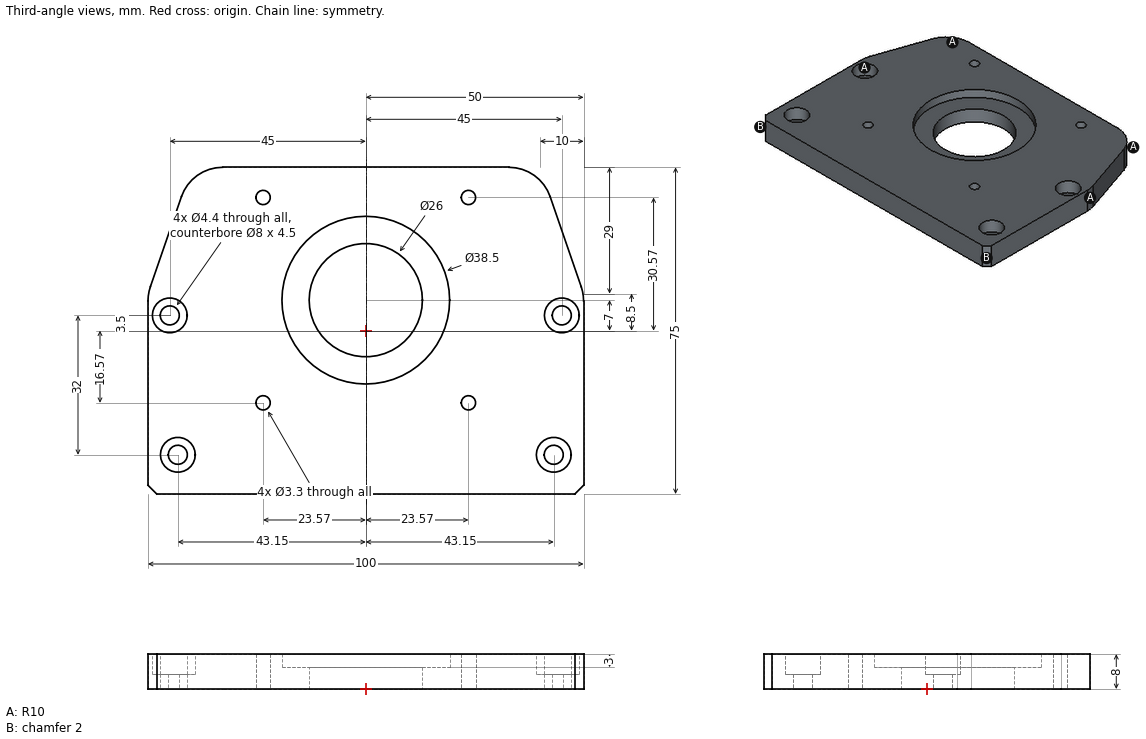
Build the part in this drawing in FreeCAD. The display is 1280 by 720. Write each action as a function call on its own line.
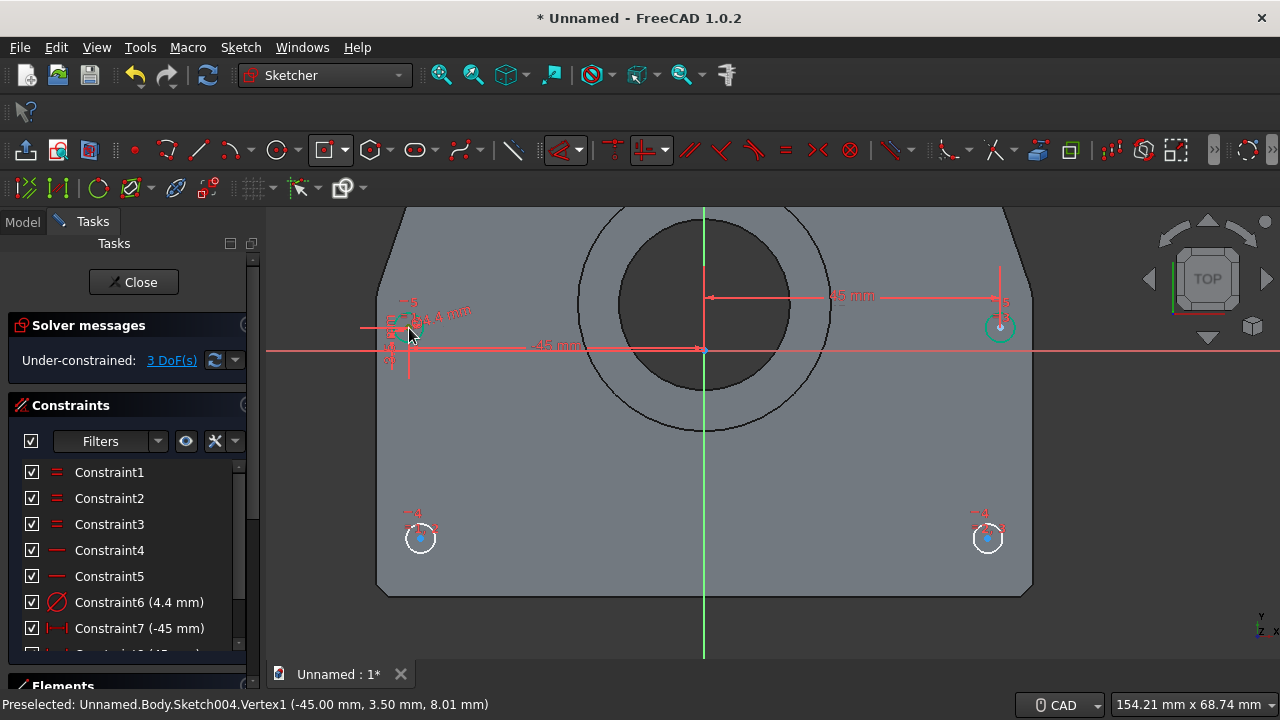
click(421, 539)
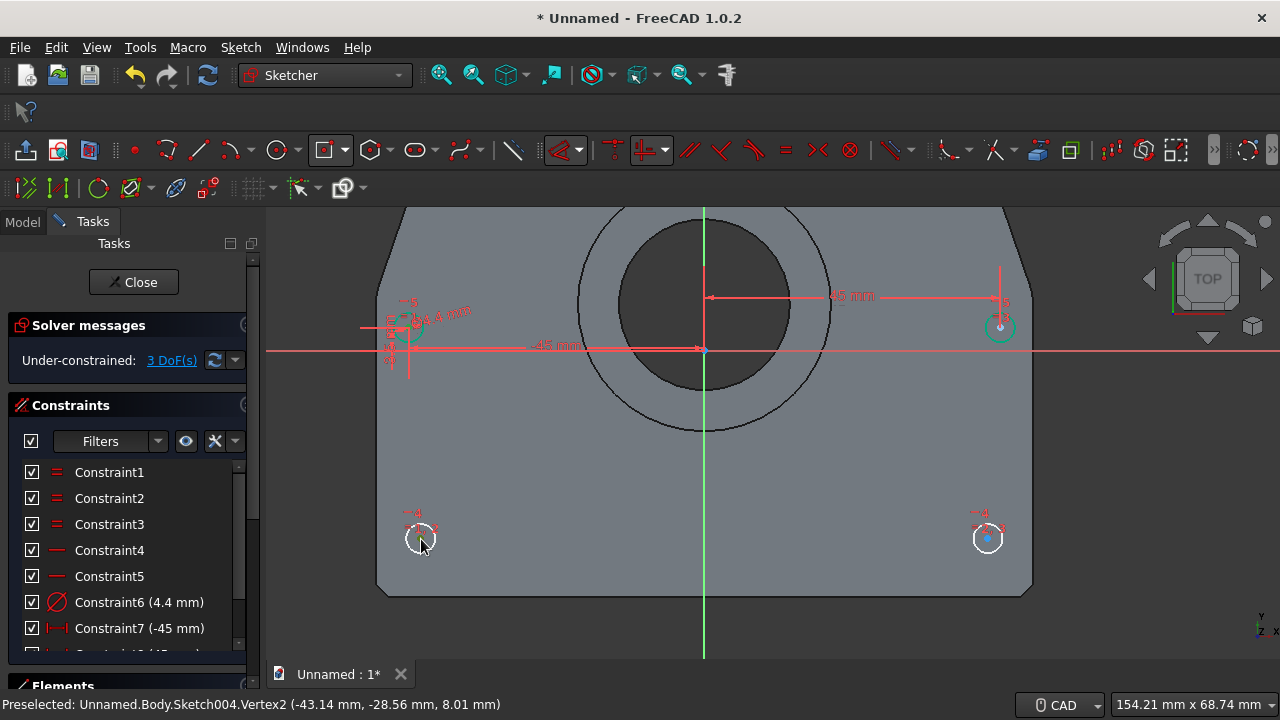
key(i)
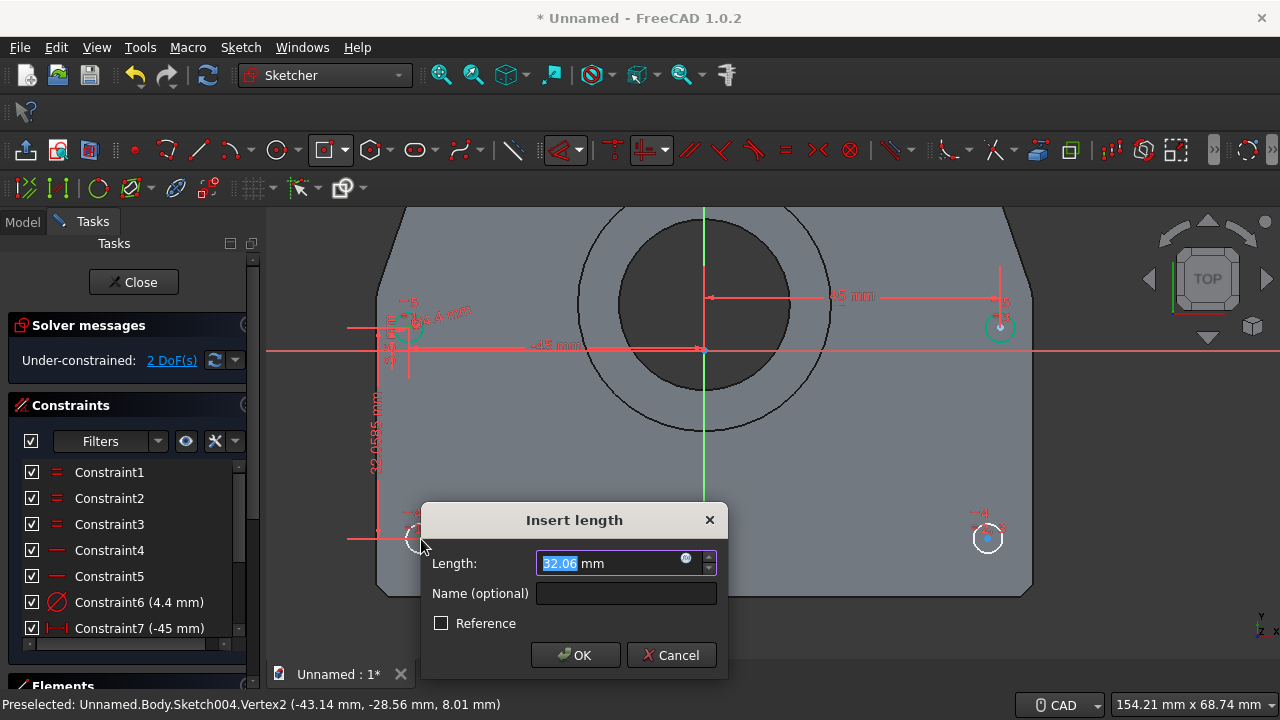
text(32)
key(Return)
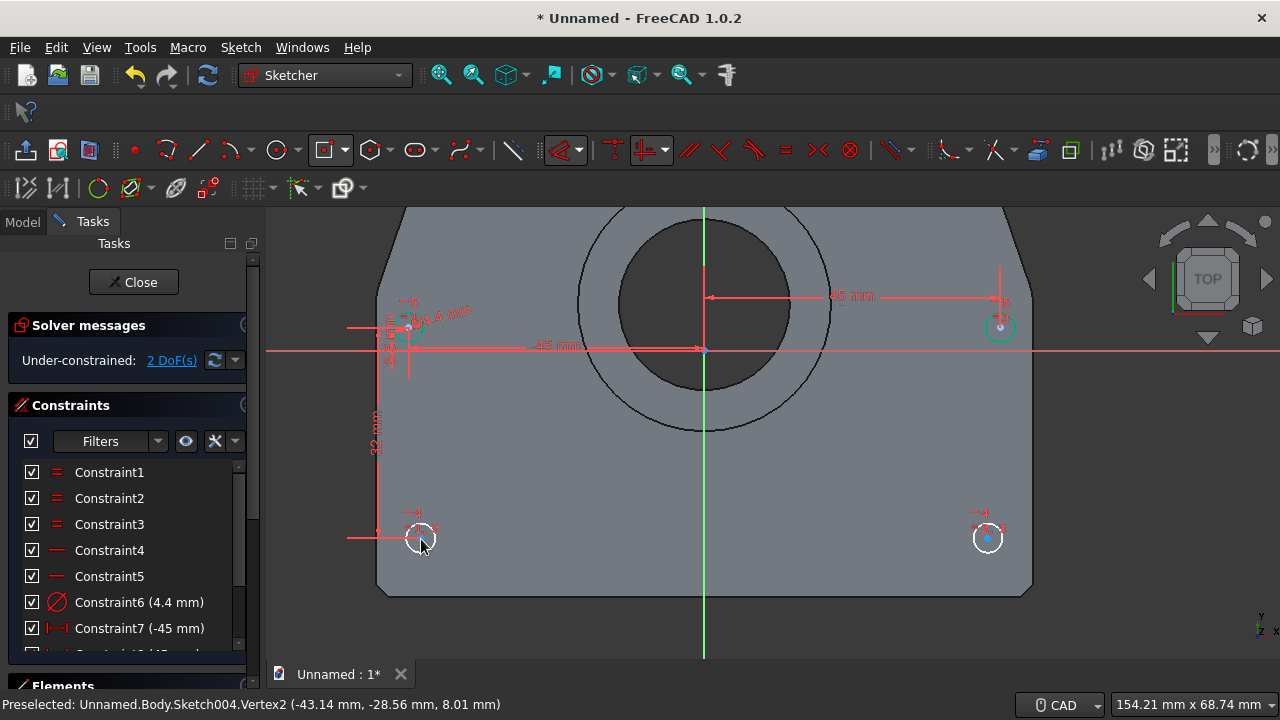
click(421, 538)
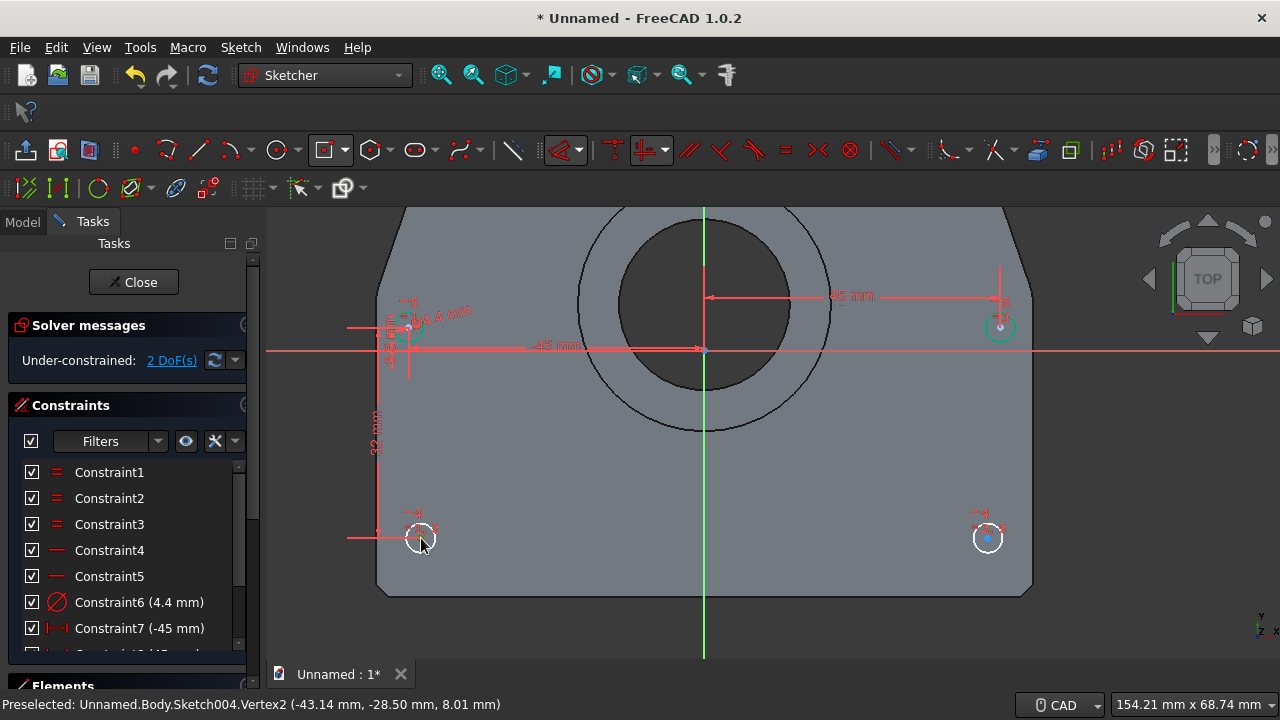
key(l)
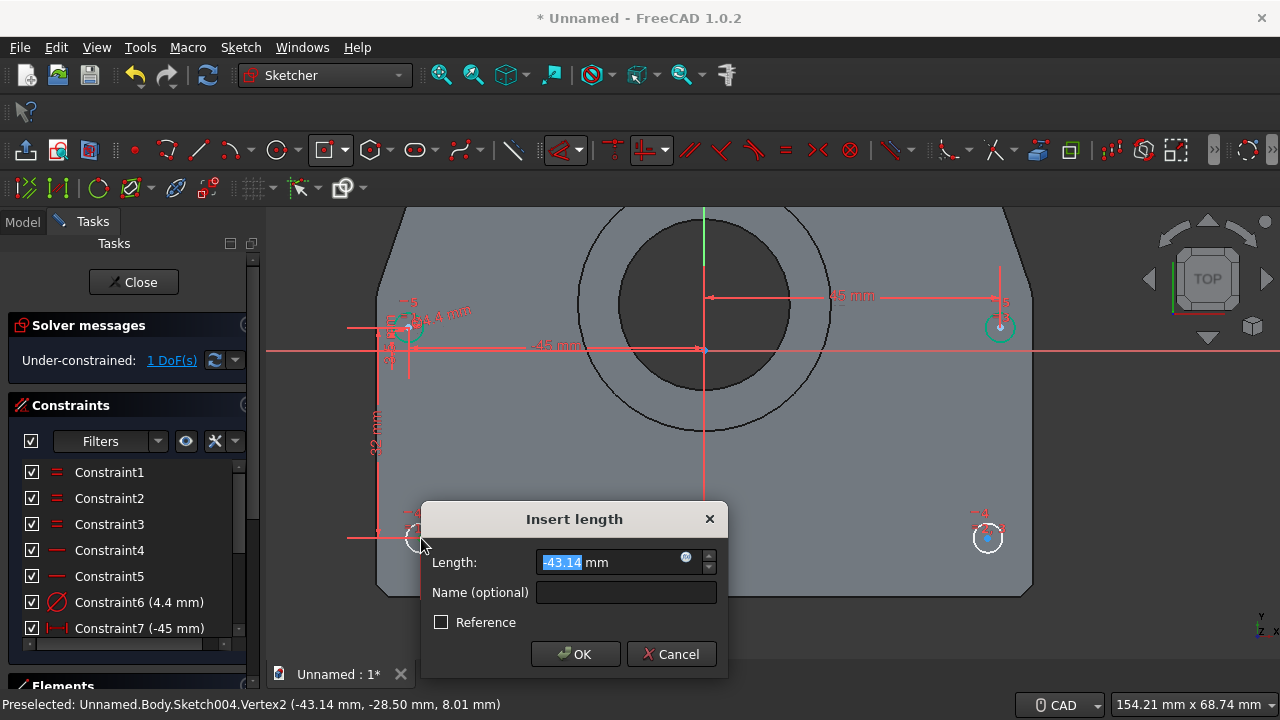
text(-43.15)
key(Return)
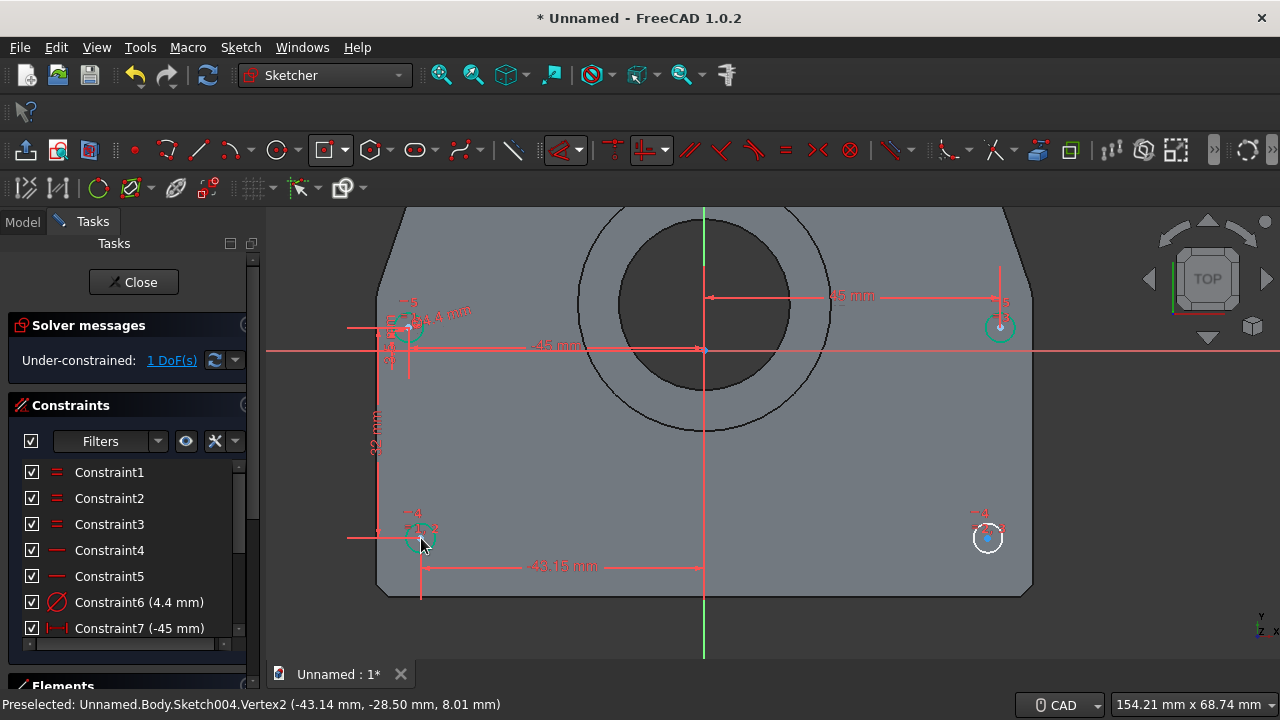
click(988, 538)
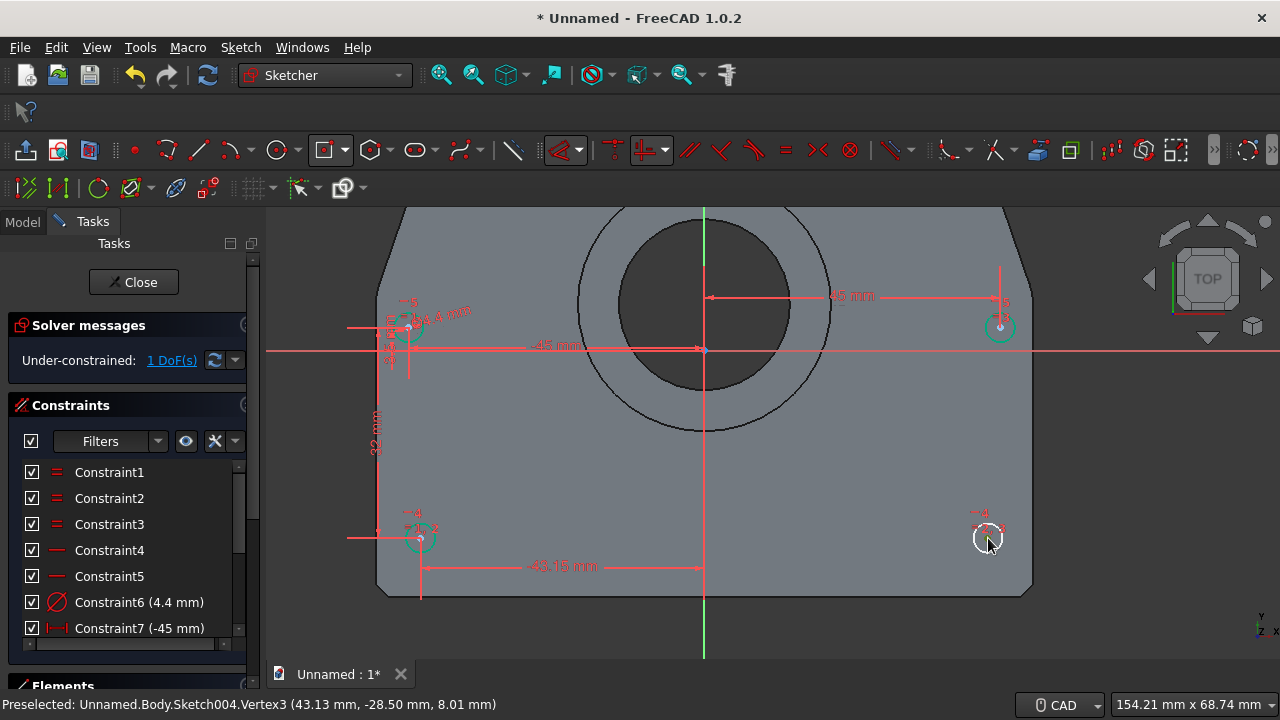
click(582, 150)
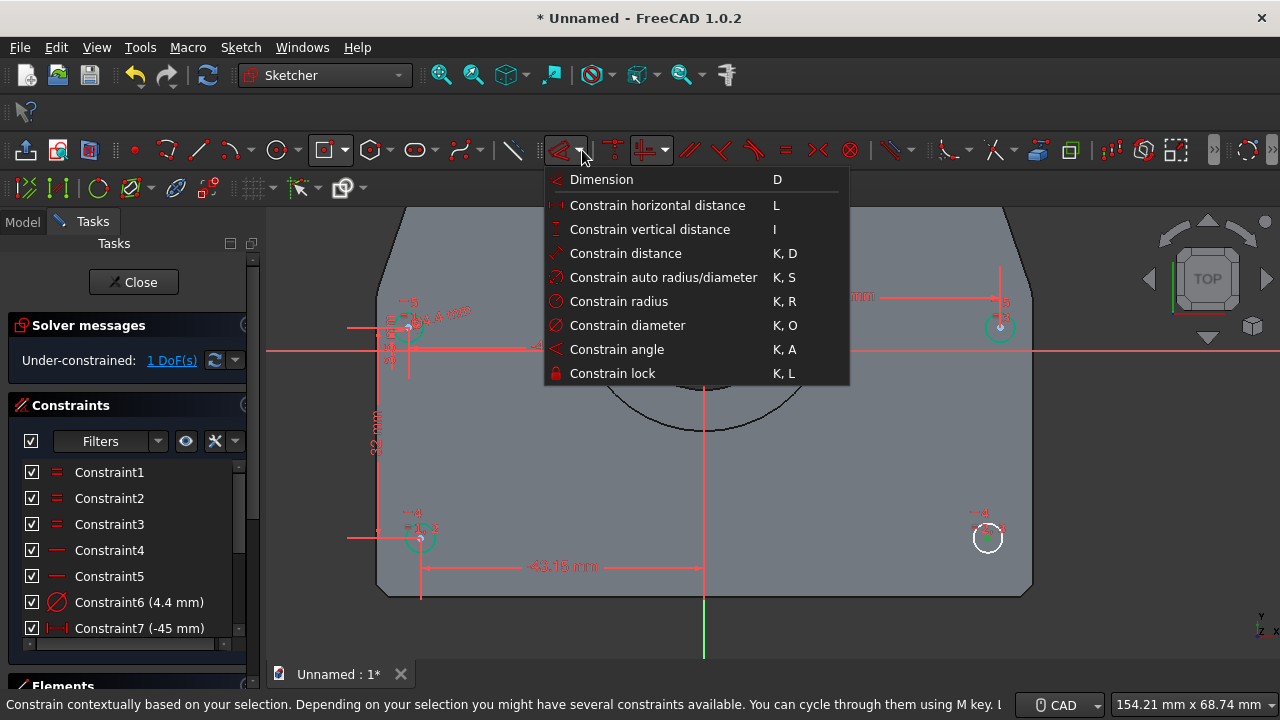
click(697, 205)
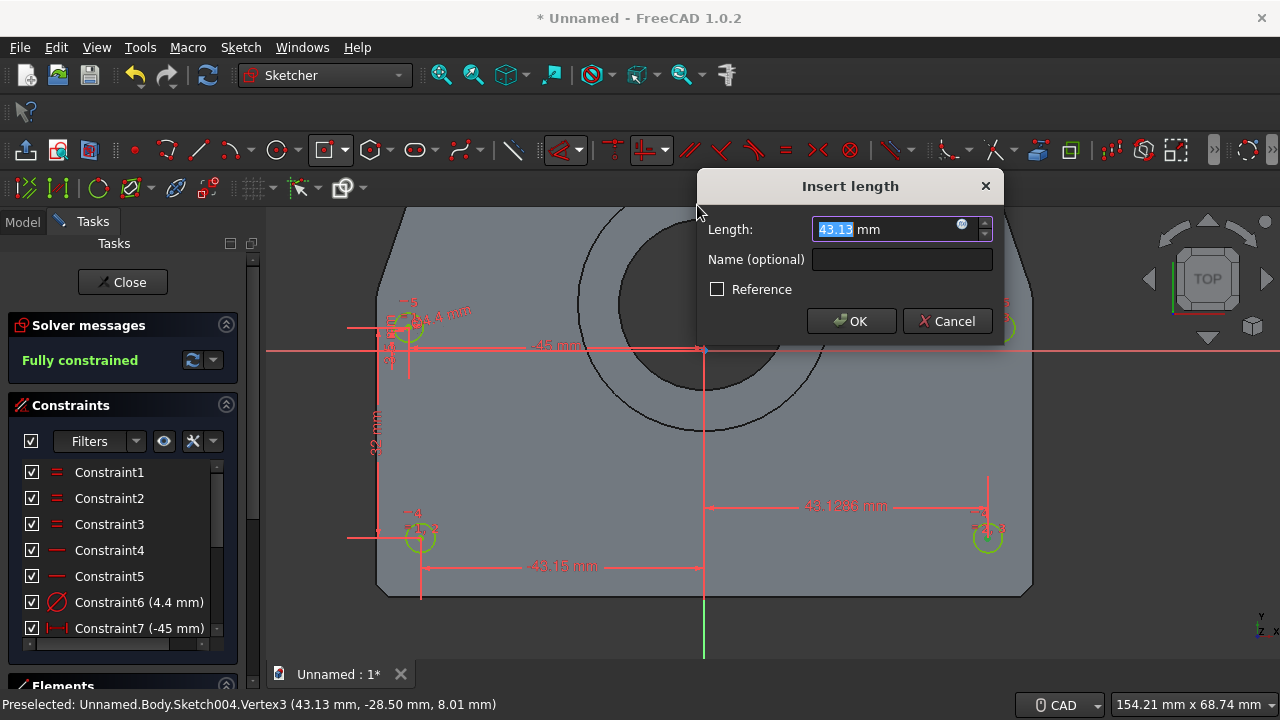
text(43.15)
key(Return)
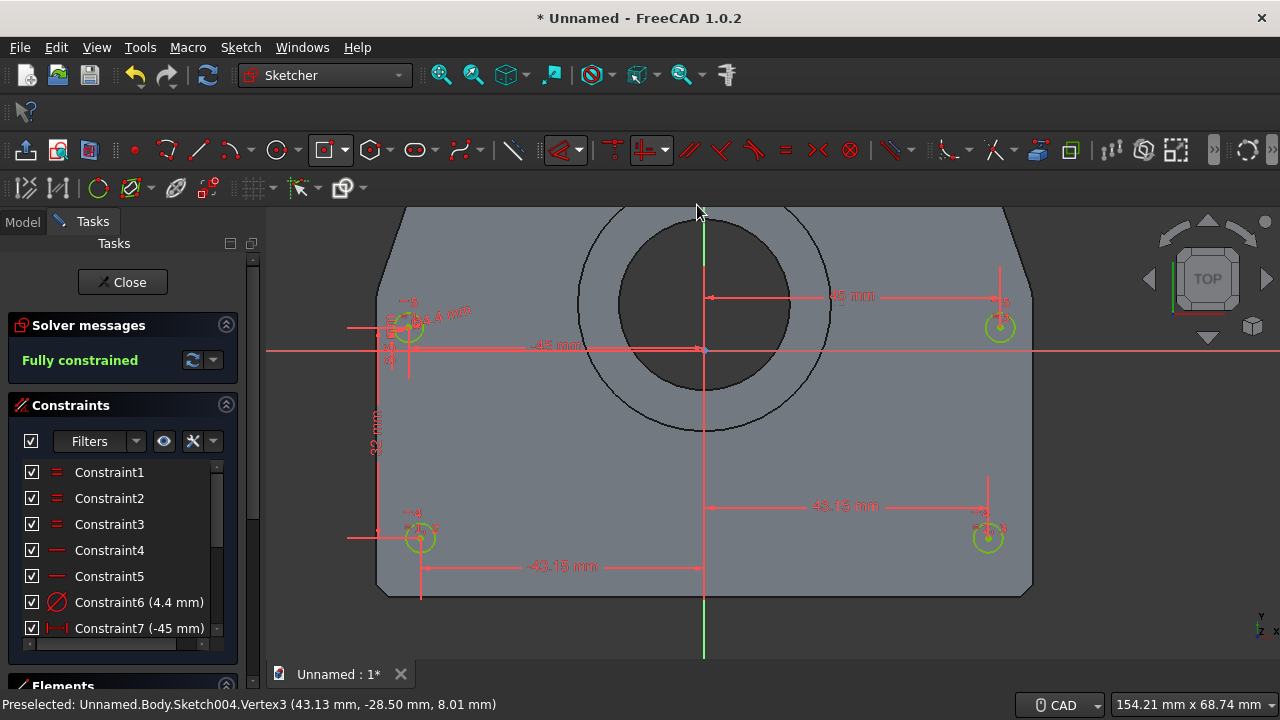
click(123, 282)